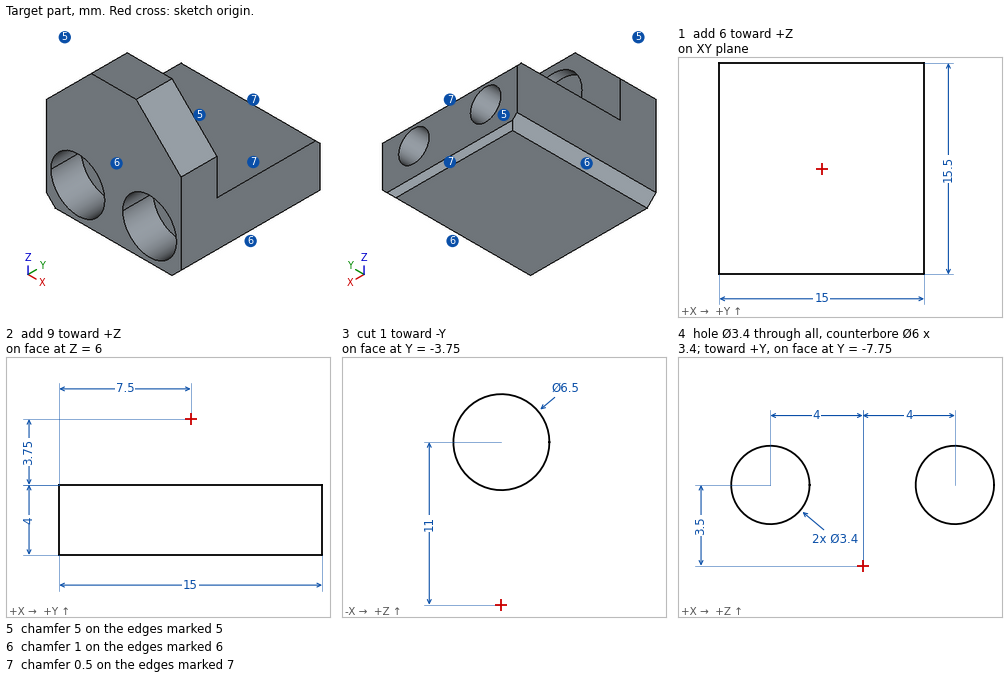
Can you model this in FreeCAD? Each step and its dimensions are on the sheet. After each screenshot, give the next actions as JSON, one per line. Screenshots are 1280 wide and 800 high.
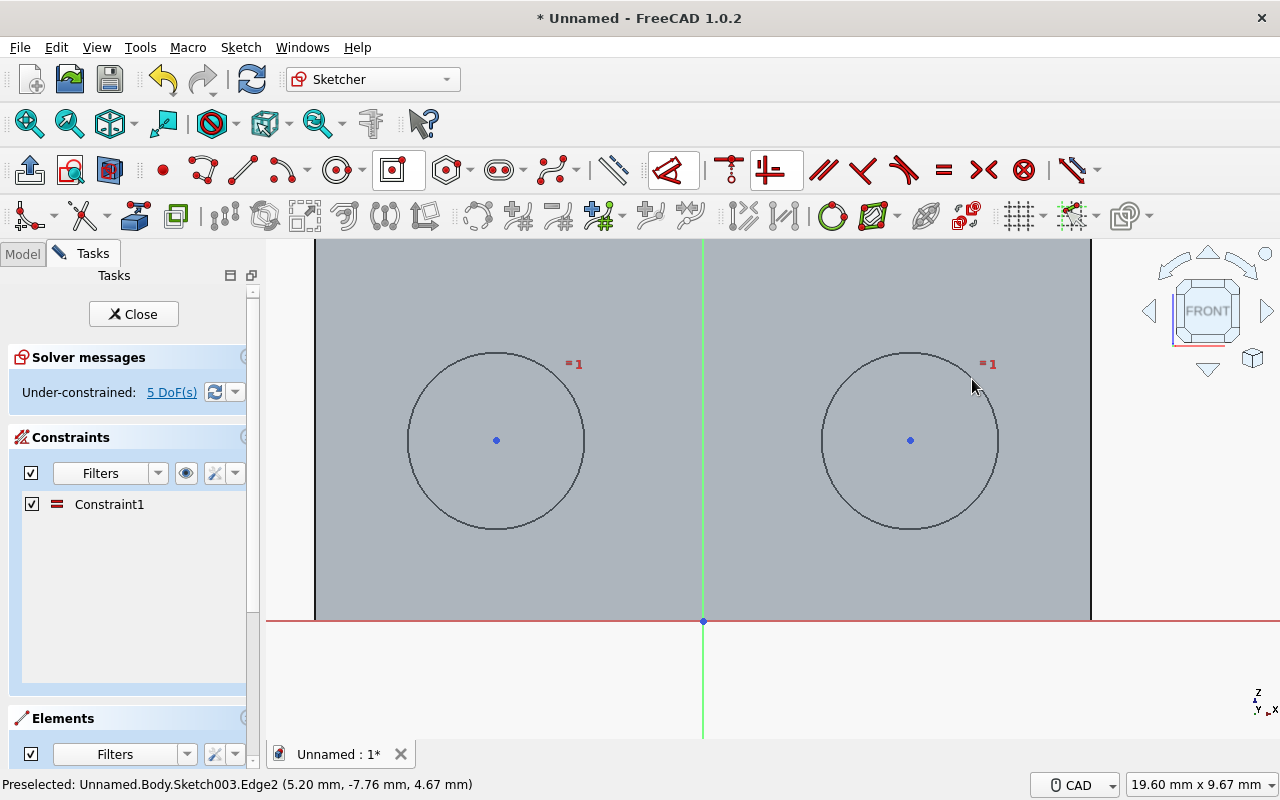
{"action": "left_click", "coordinate": [496, 441]}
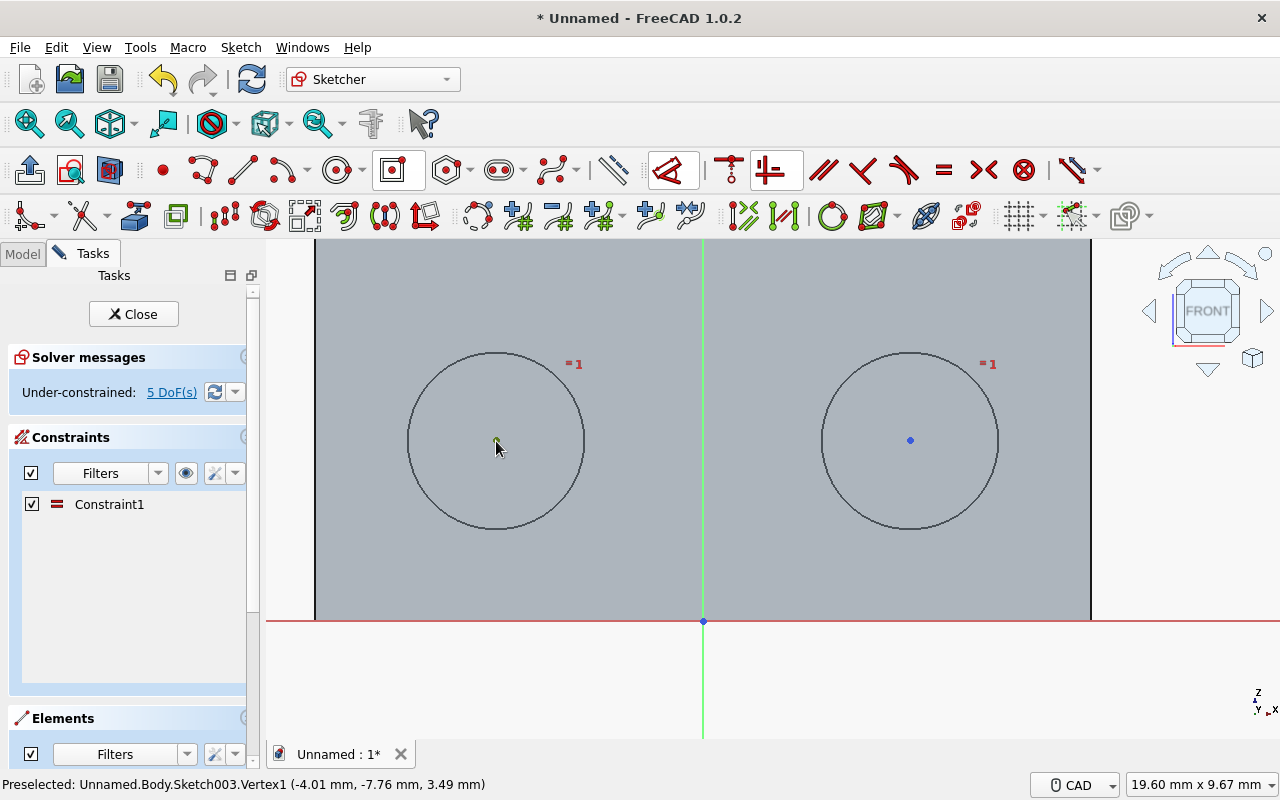
{"action": "left_click", "coordinate": [910, 441]}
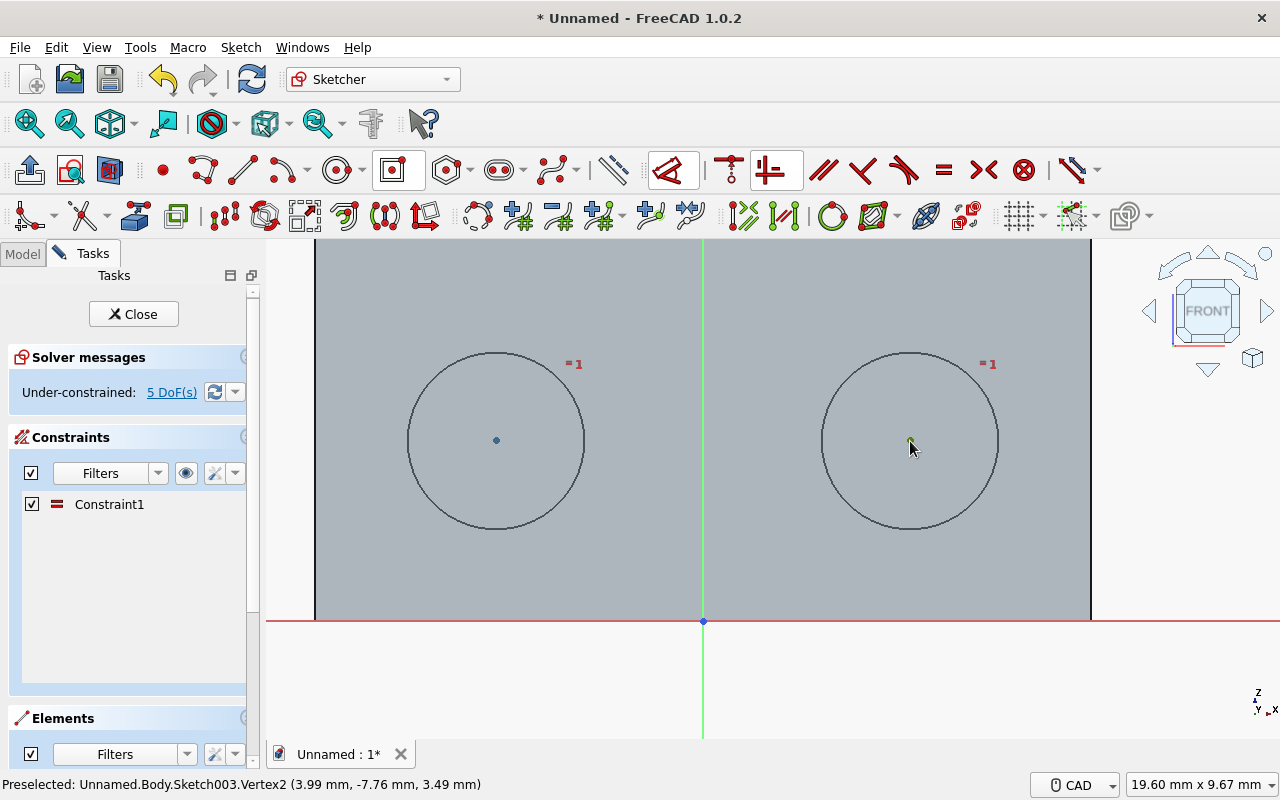
{"action": "key", "text": "h"}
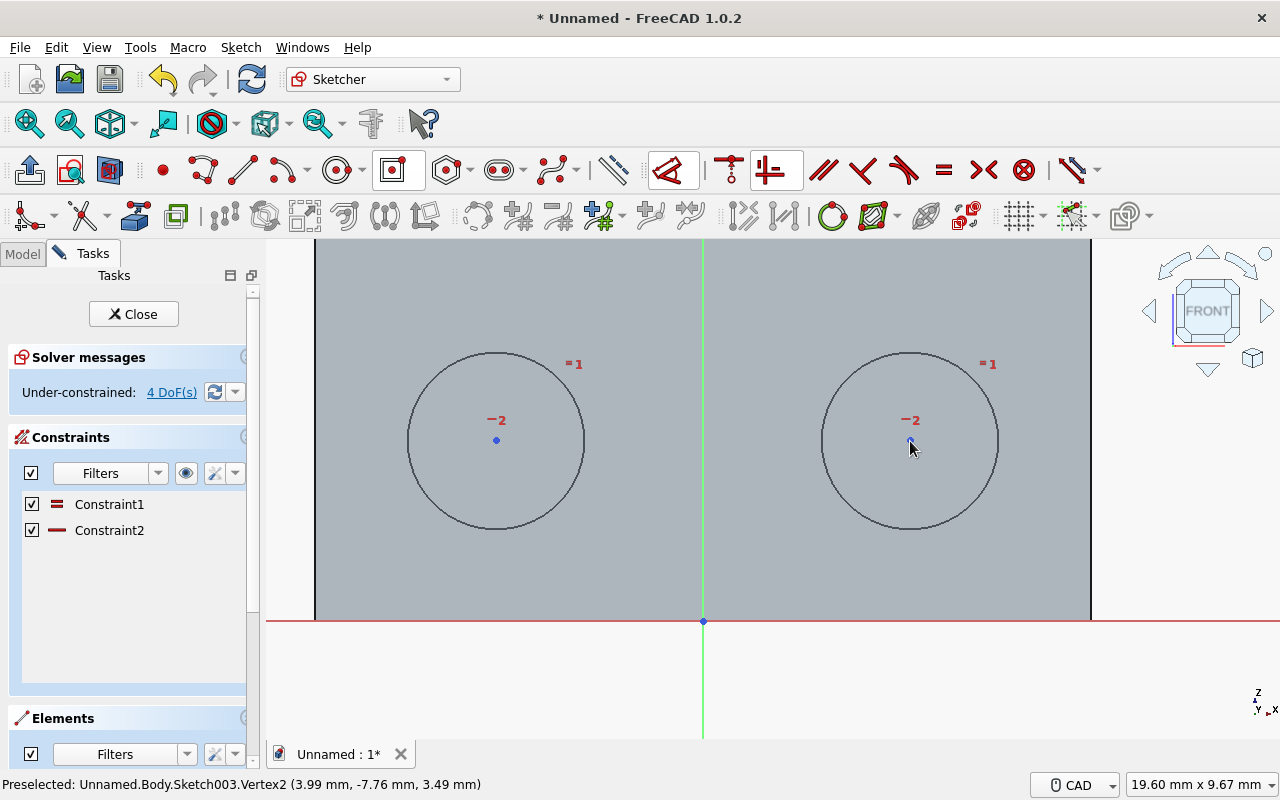
{"action": "left_click", "coordinate": [668, 170]}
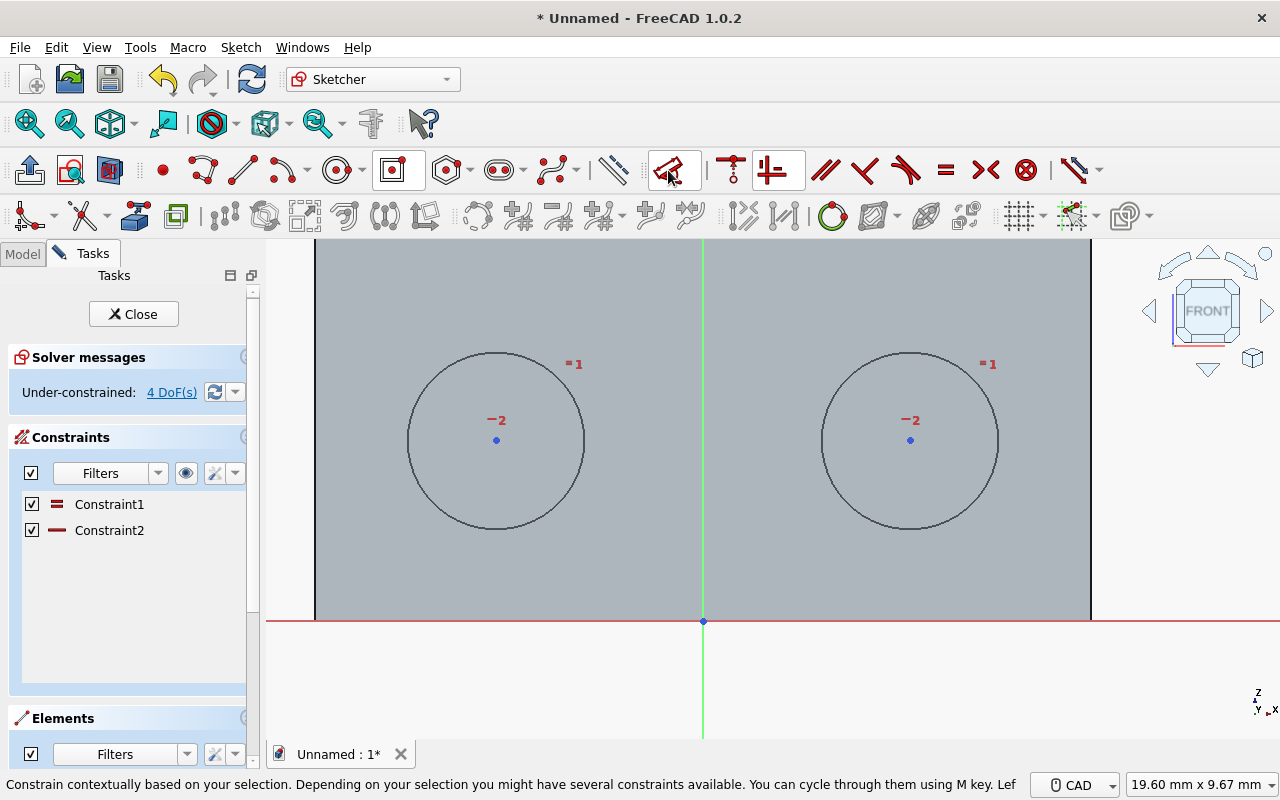
{"action": "left_click", "coordinate": [558, 378]}
{"action": "left_click", "coordinate": [580, 355]}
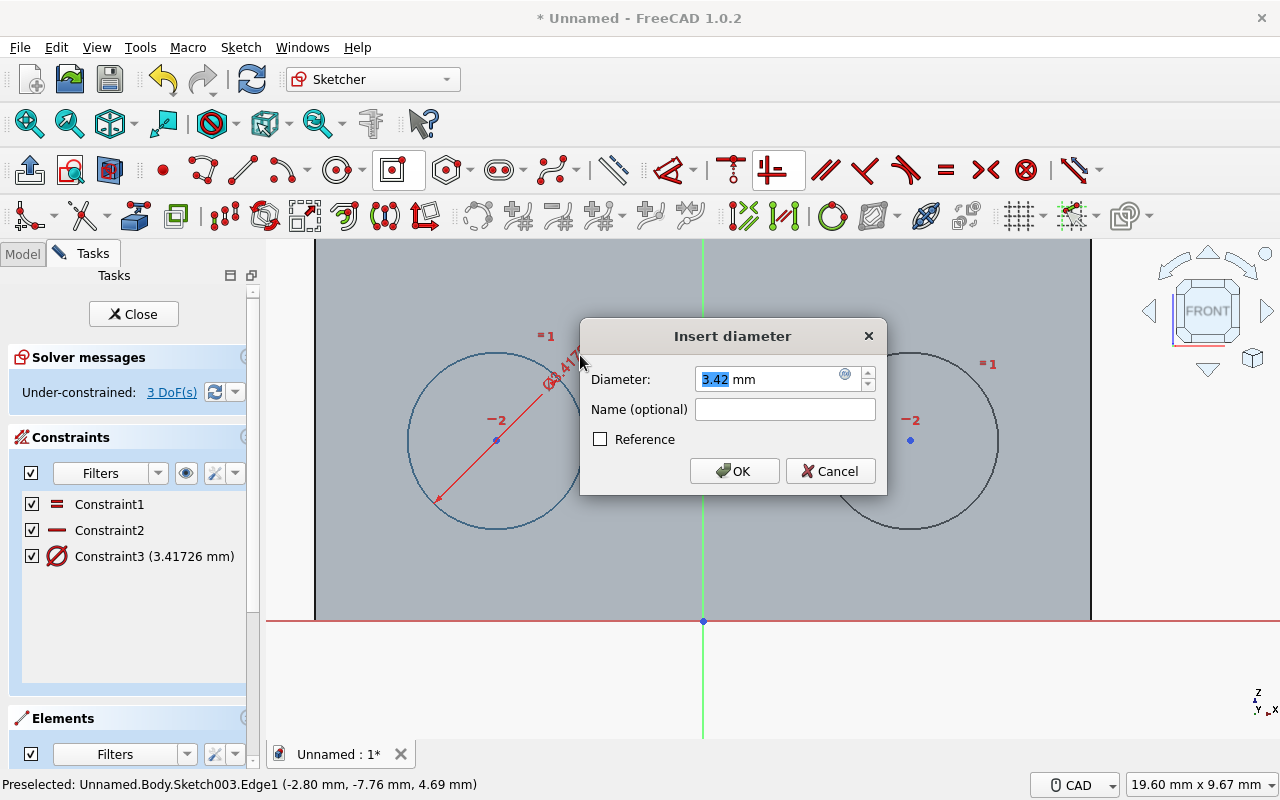
{"action": "type", "text": "3.4"}
{"action": "key", "text": "Return"}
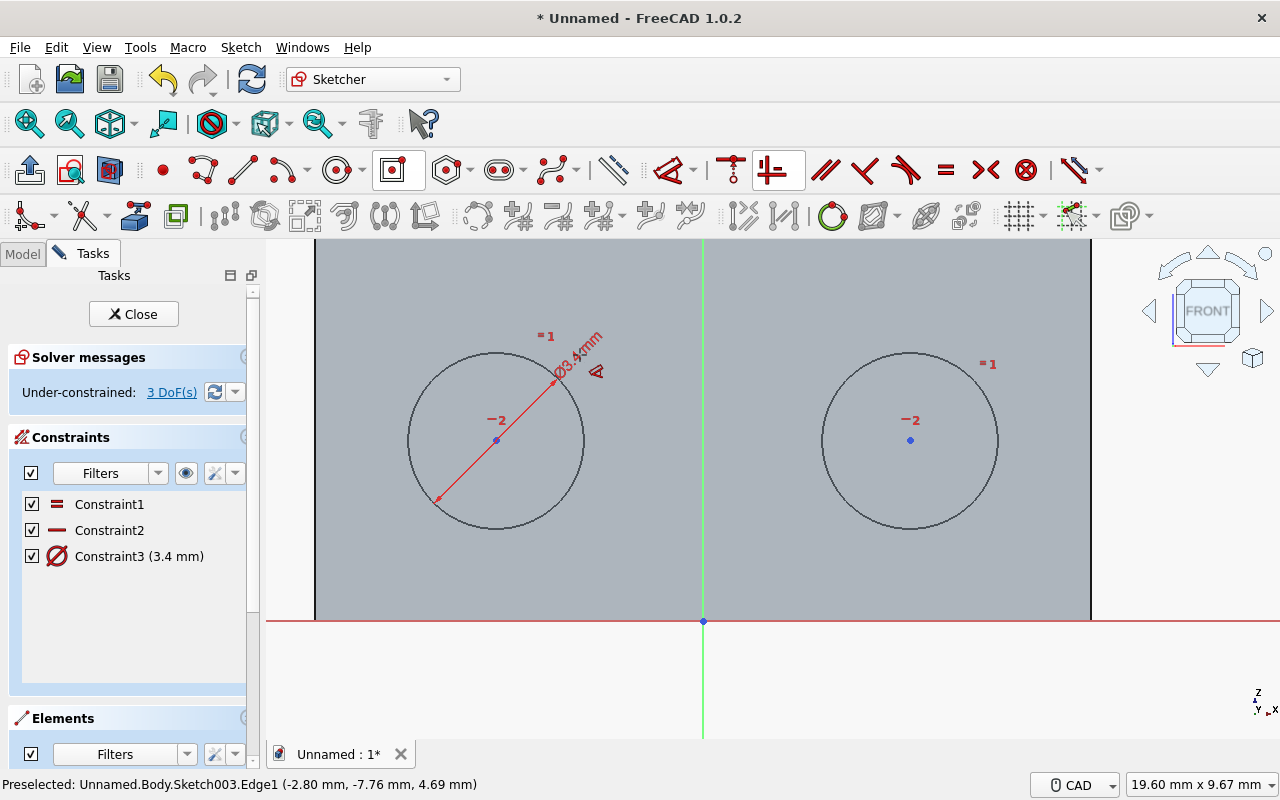
{"action": "left_click", "coordinate": [496, 441]}
{"action": "left_click", "coordinate": [600, 655]}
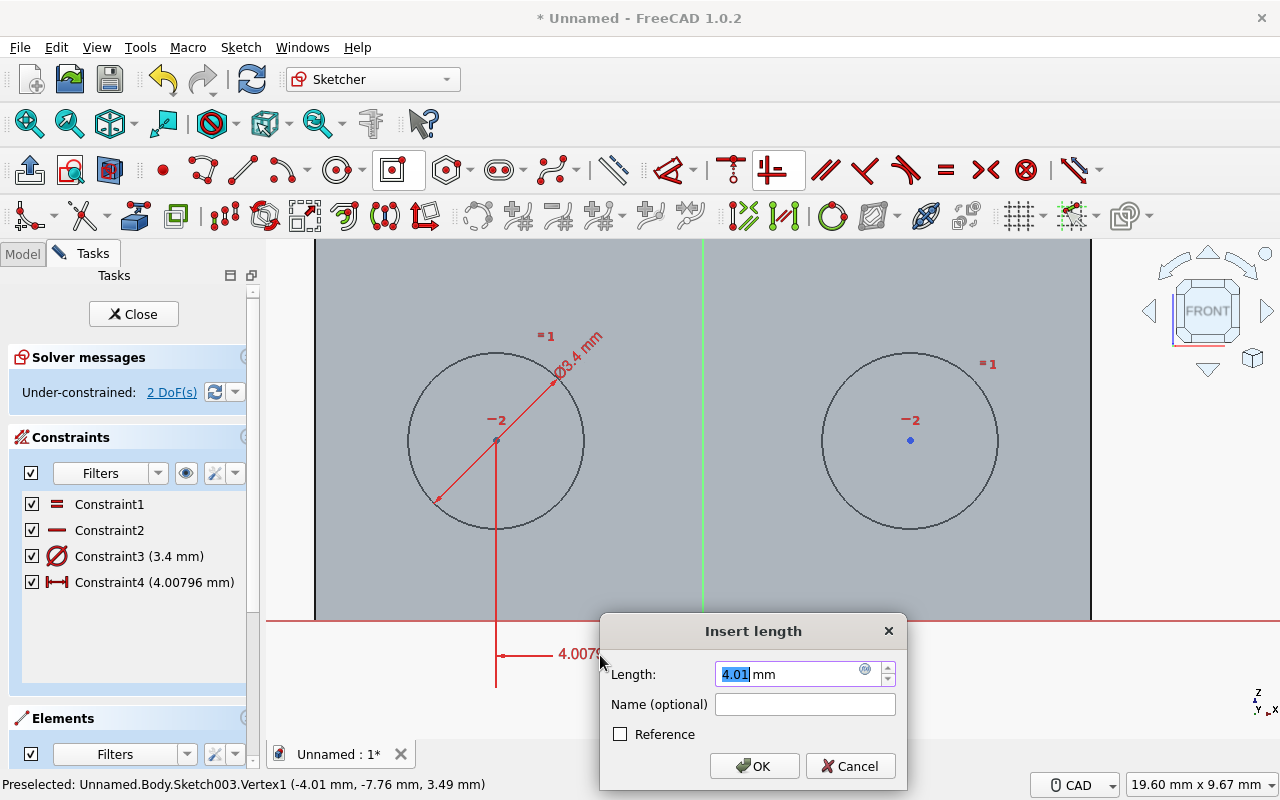
{"action": "type", "text": "4"}
{"action": "key", "text": "Return"}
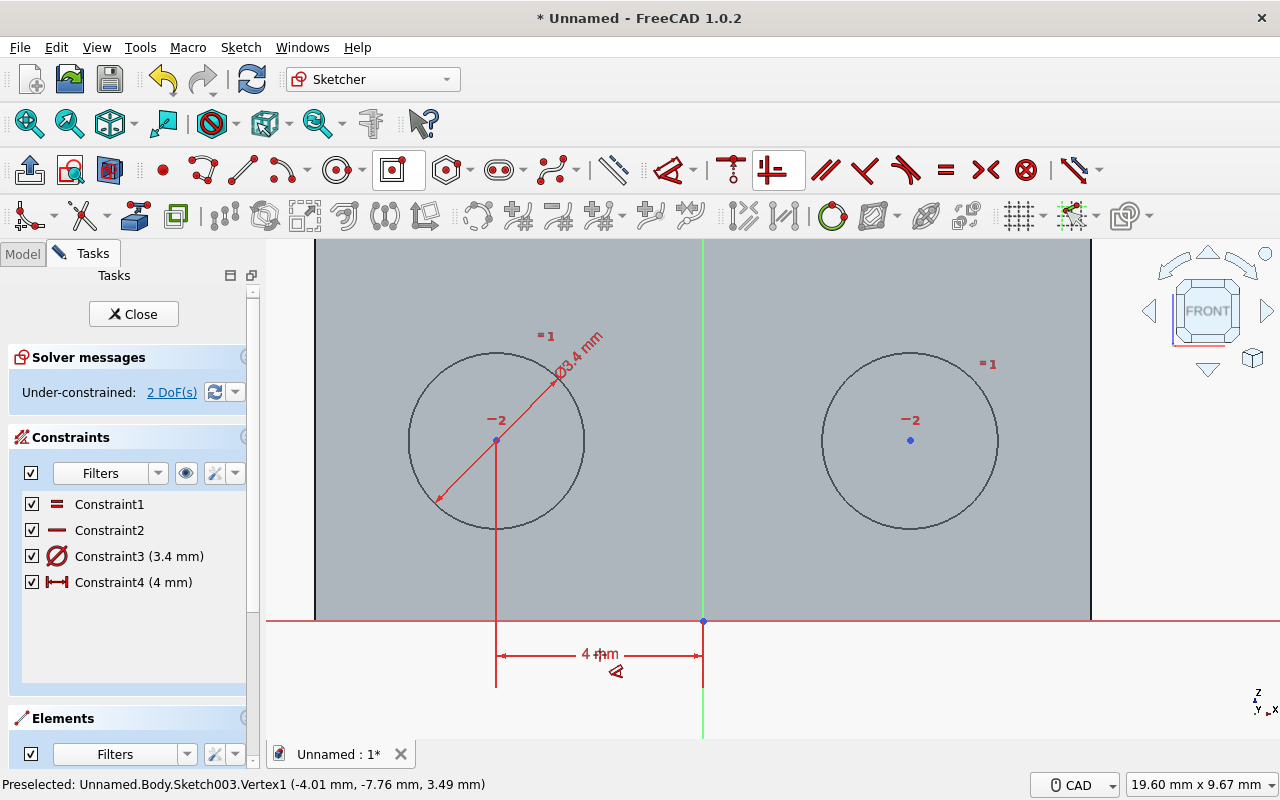
{"action": "left_click", "coordinate": [910, 441]}
{"action": "left_click", "coordinate": [807, 655]}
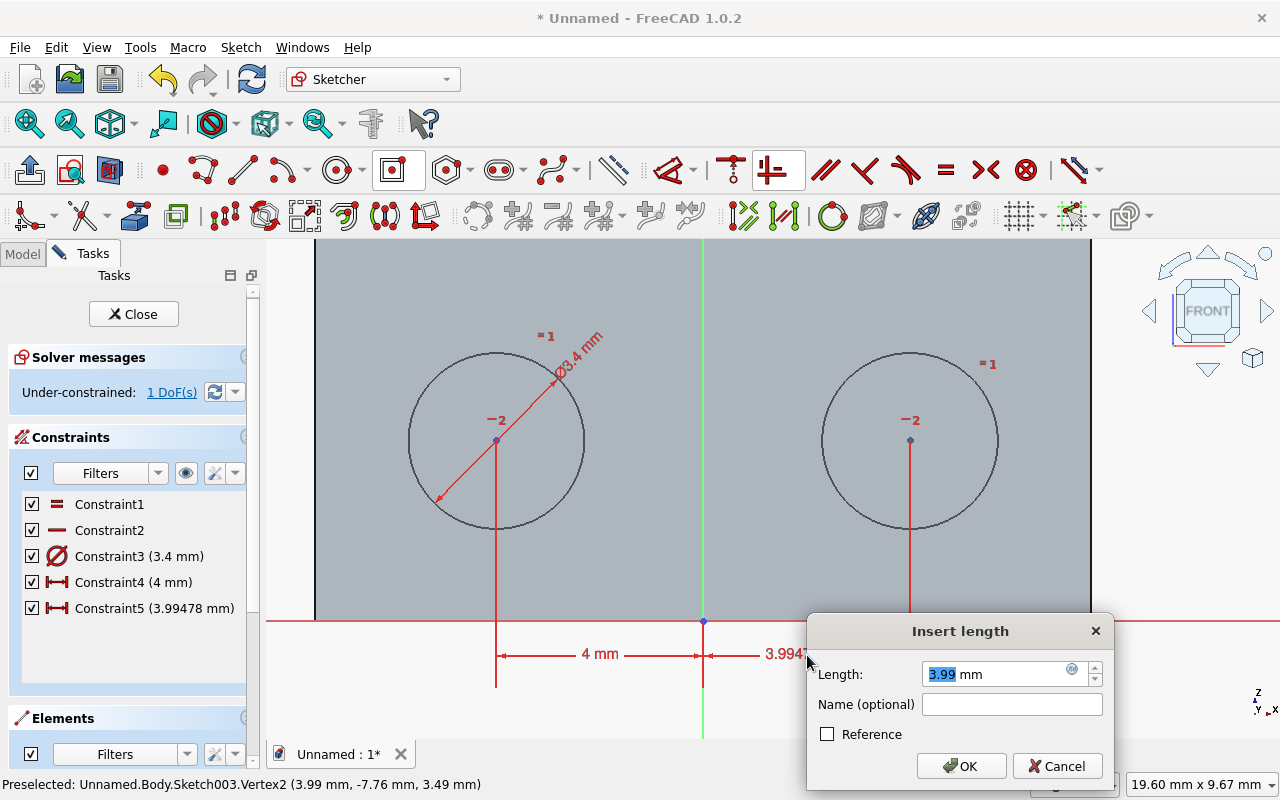
{"action": "type", "text": "4"}
{"action": "key", "text": "Return"}